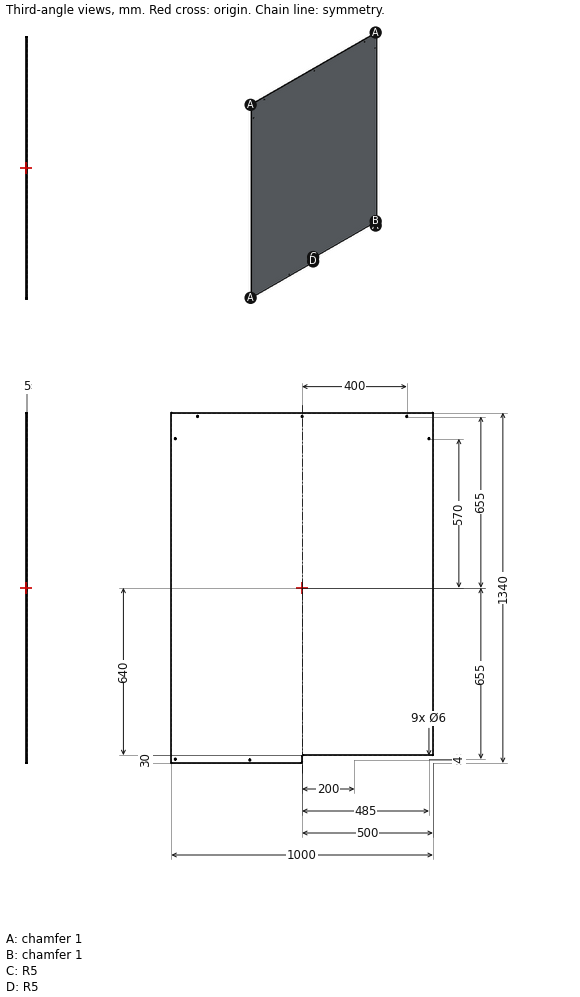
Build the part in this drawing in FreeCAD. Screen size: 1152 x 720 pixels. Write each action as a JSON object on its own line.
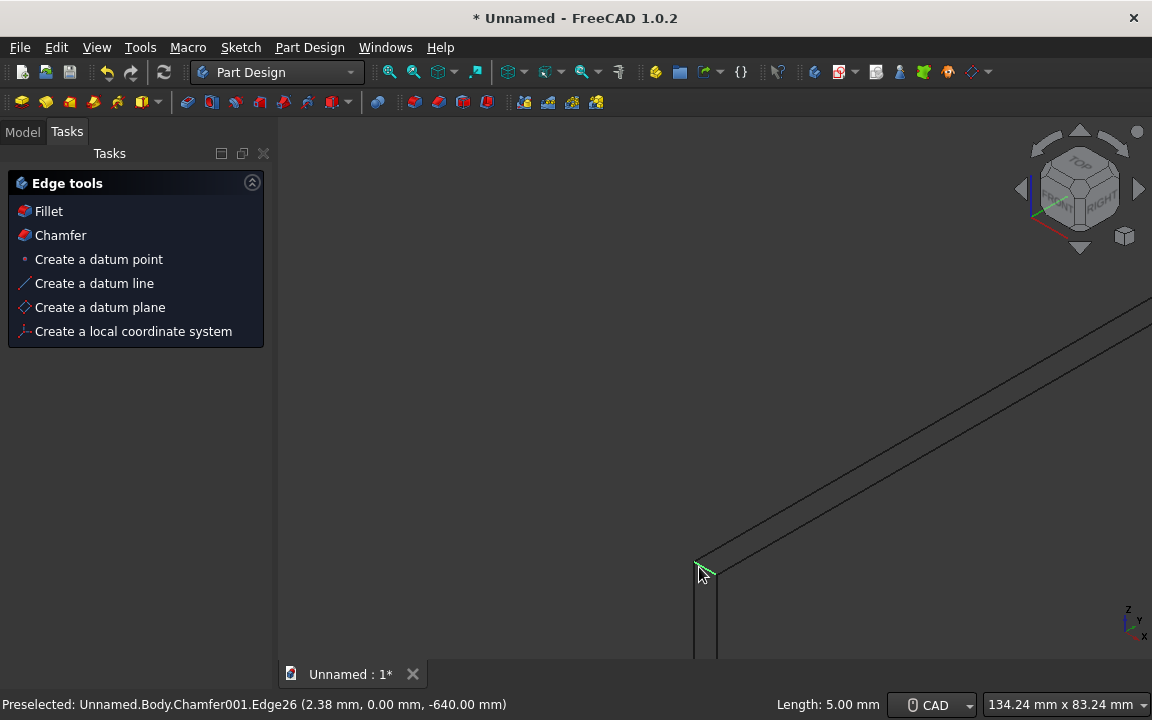
{"action": "key", "text": "v 1"}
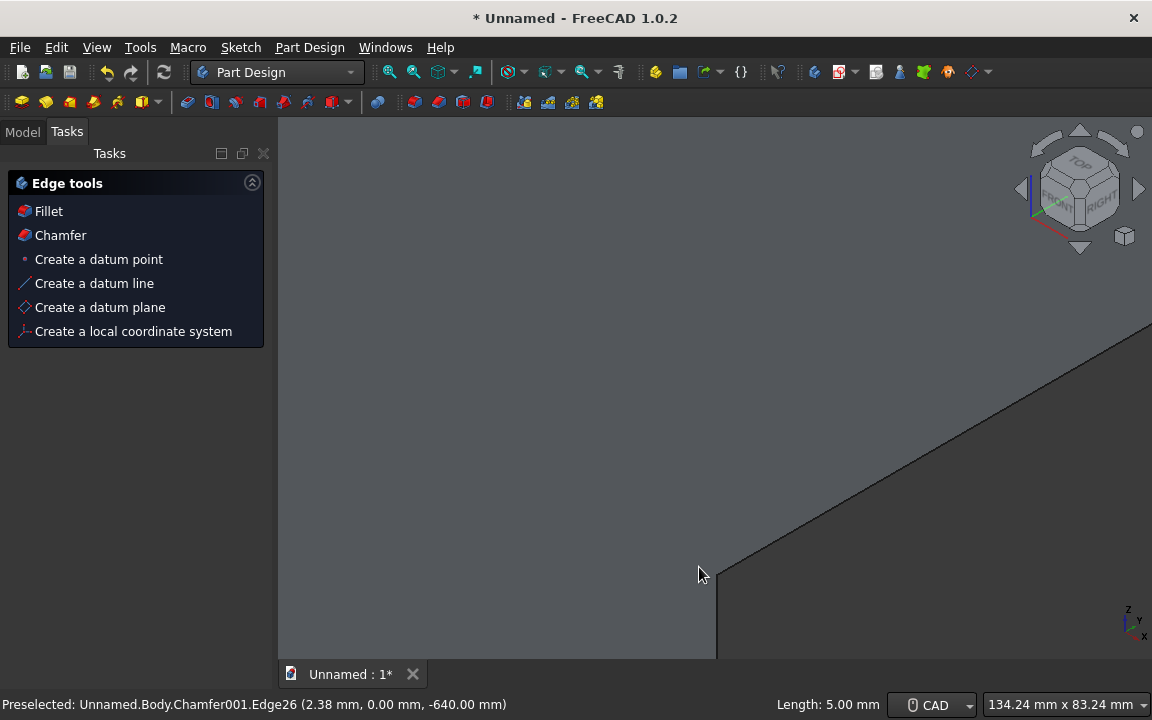
{"action": "left_click", "coordinate": [416, 102]}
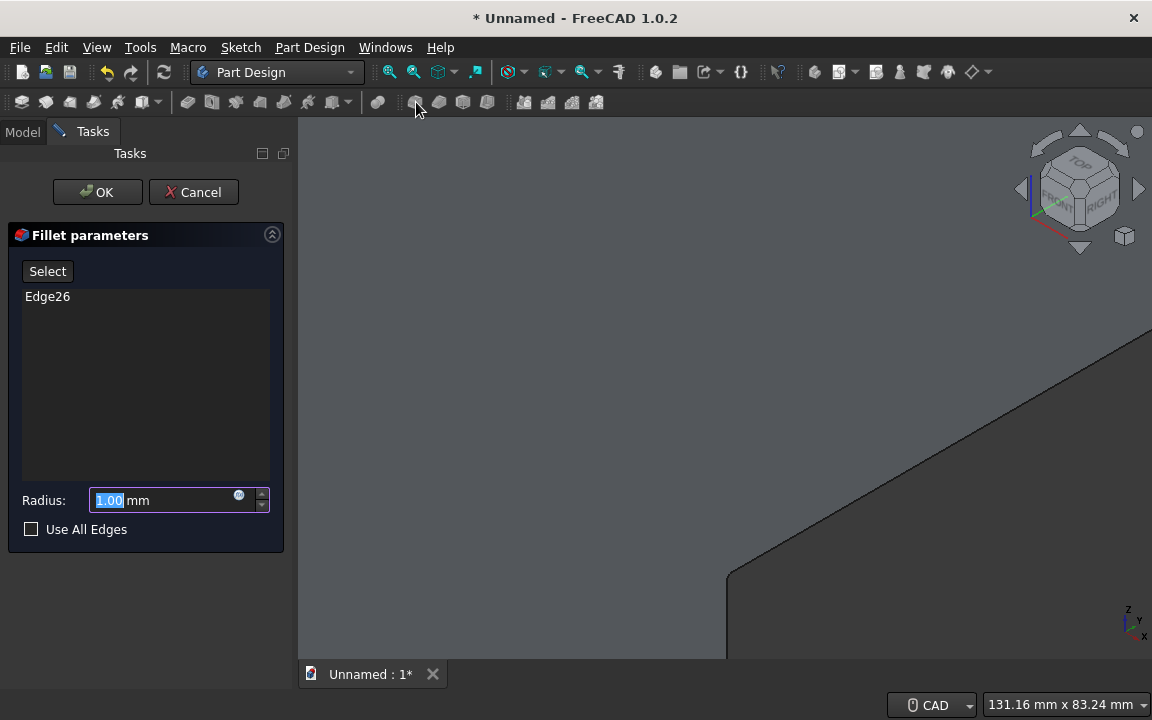
{"action": "type", "text": "5"}
{"action": "key", "text": "Tab"}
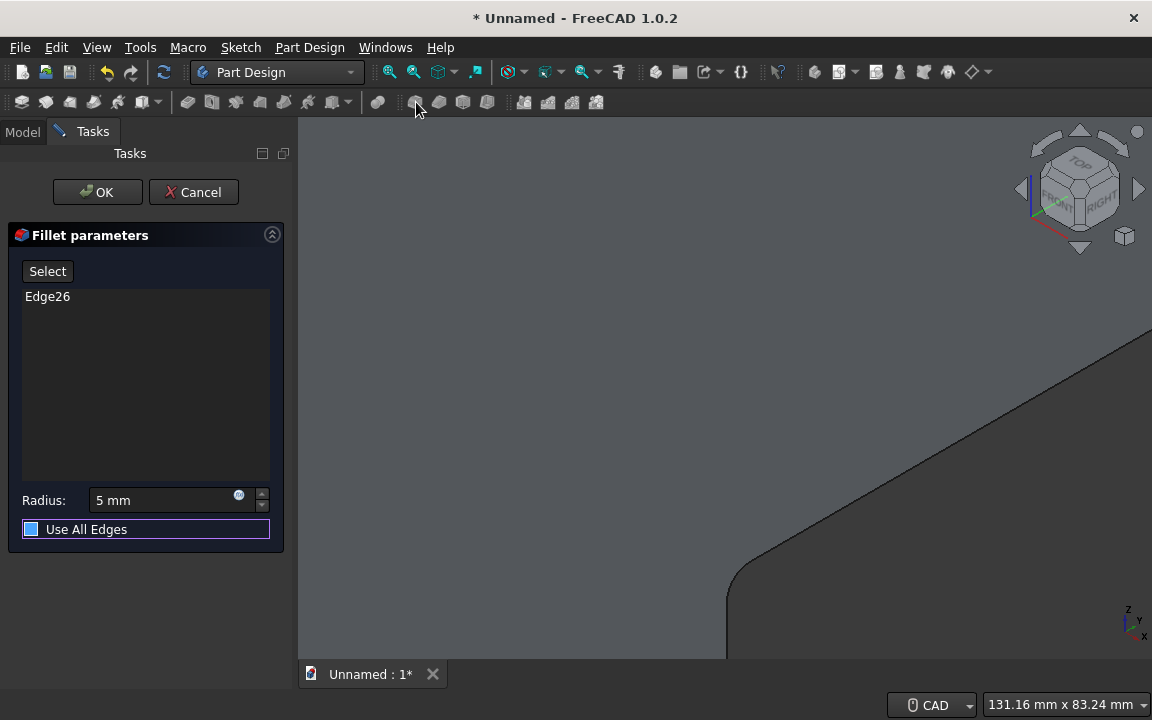
{"action": "left_click", "coordinate": [98, 192]}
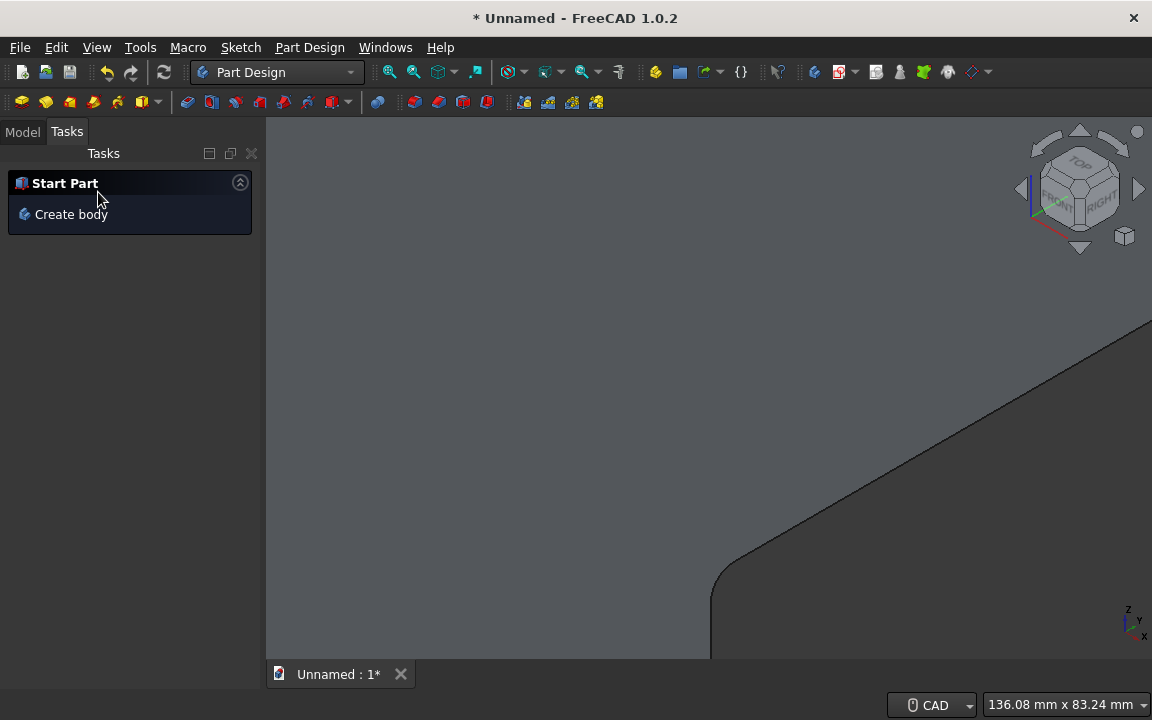
{"action": "left_click", "coordinate": [390, 72]}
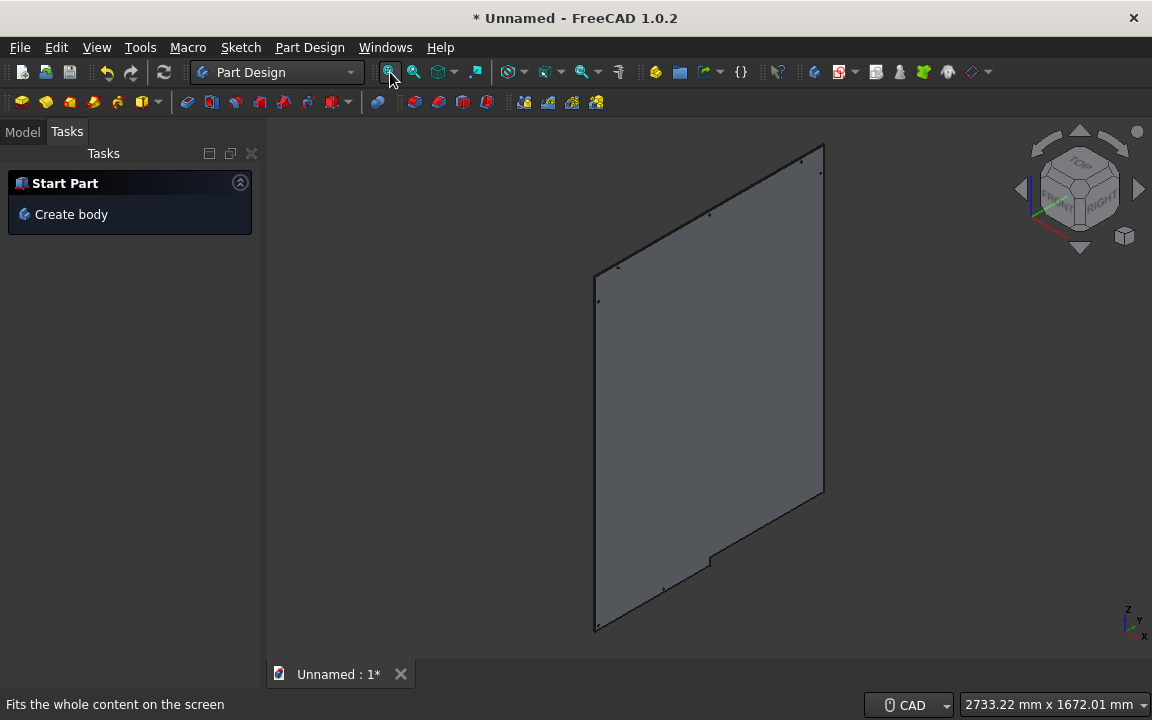
{"action": "scroll", "coordinate": [709, 564], "scroll_direction": "up", "scroll_amount": 15}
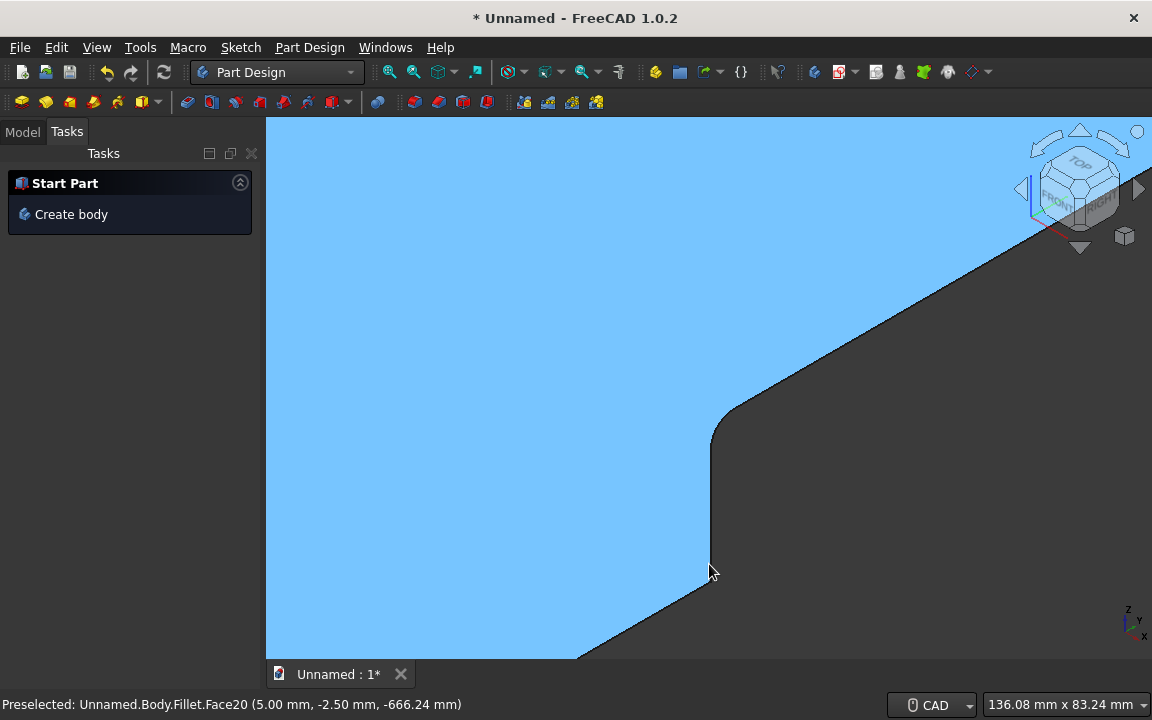
{"action": "left_click", "coordinate": [390, 72]}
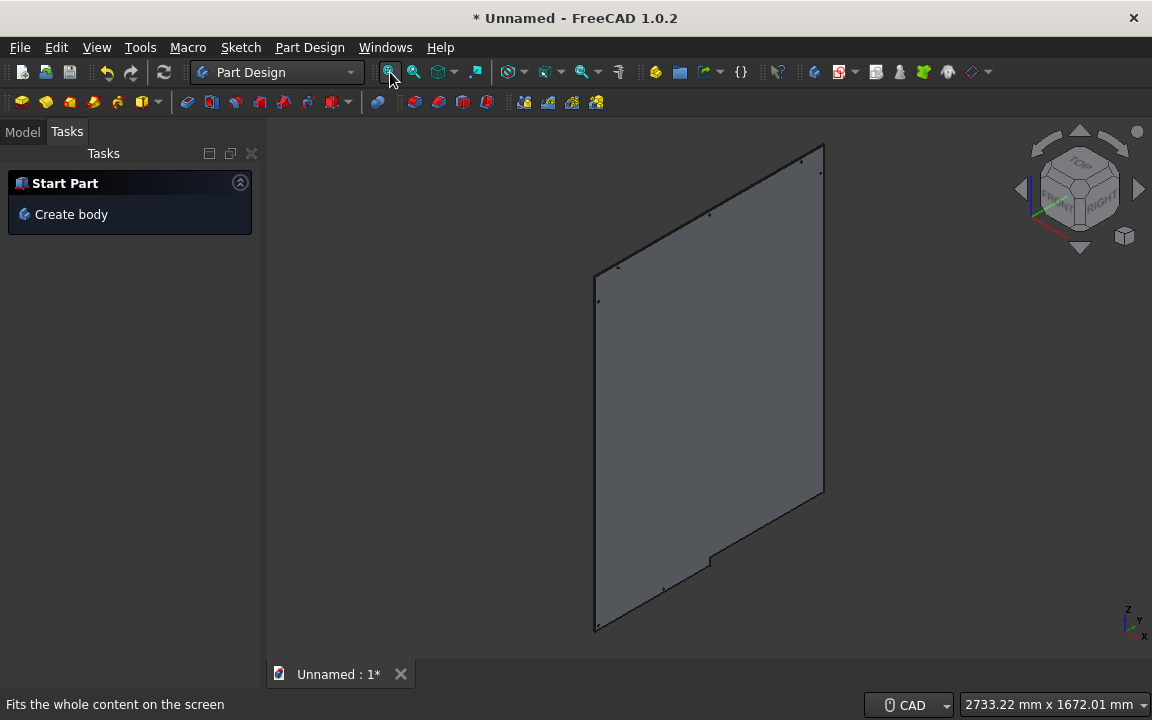
{"action": "key", "text": "2"}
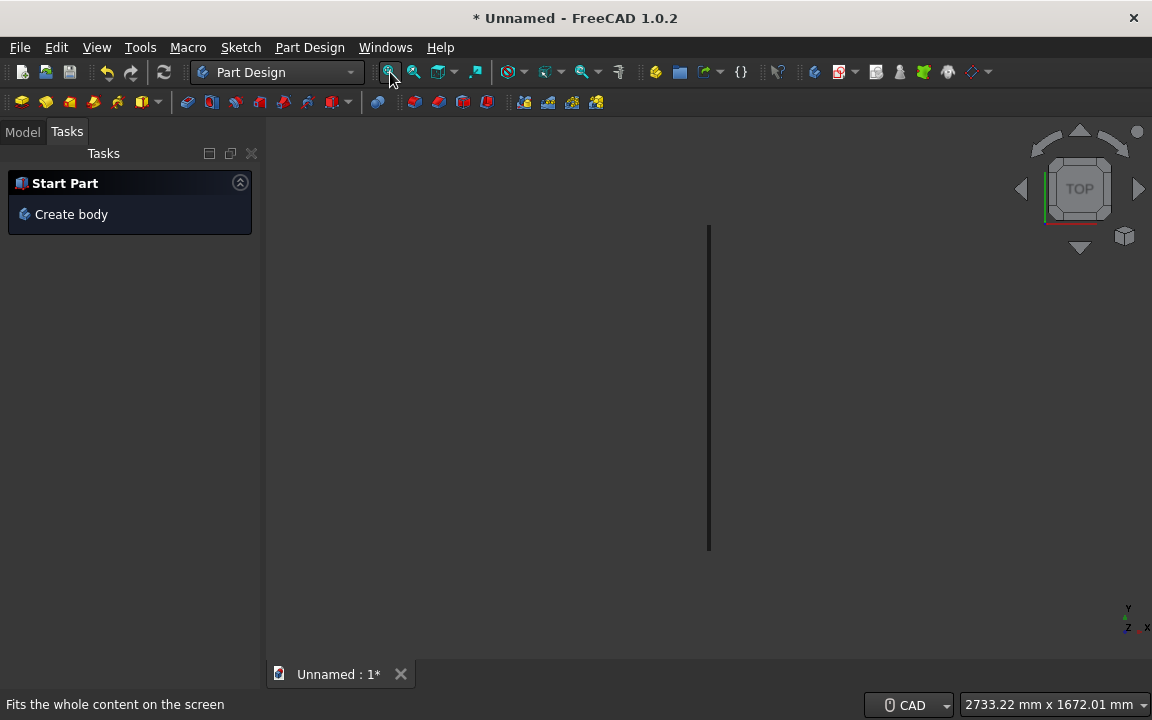
{"action": "scroll", "coordinate": [709, 387], "scroll_direction": "up", "scroll_amount": 15}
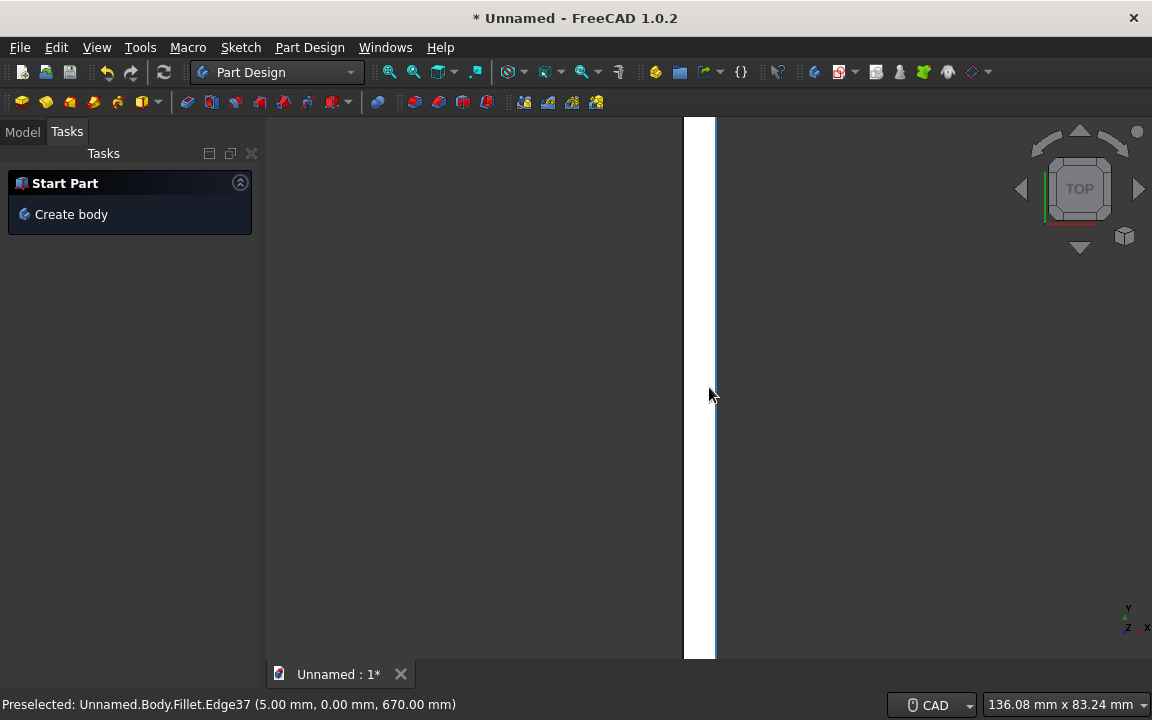
{"action": "left_click", "coordinate": [390, 72]}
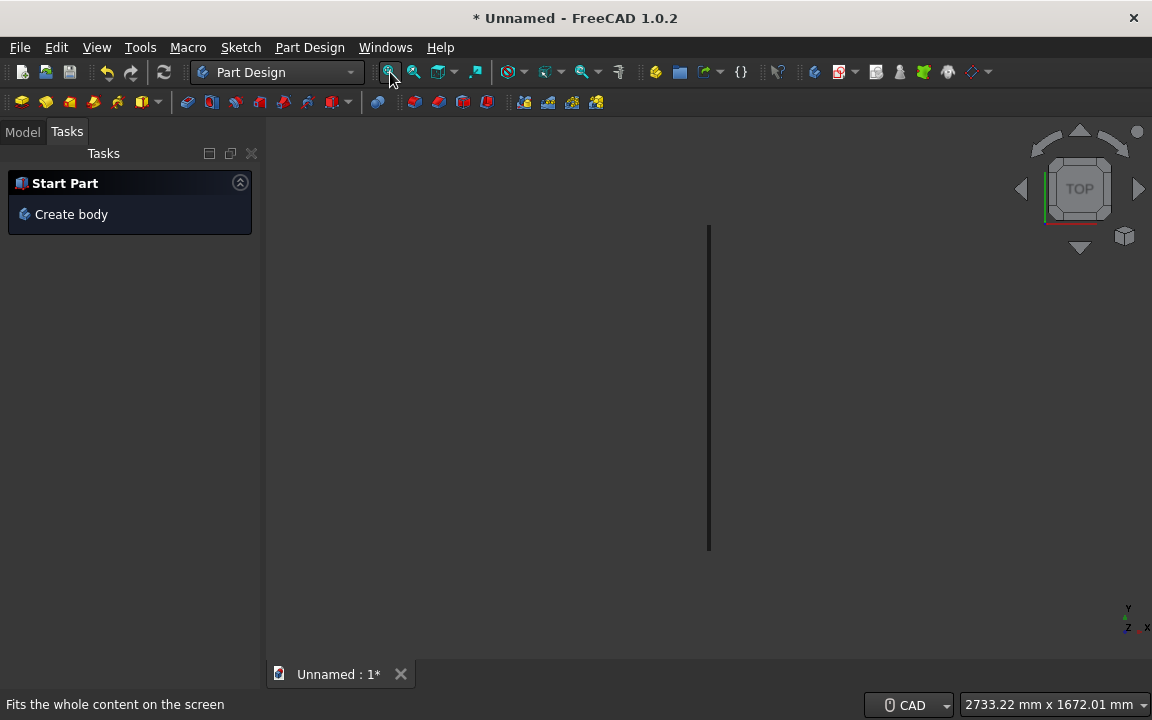
{"action": "key", "text": "0"}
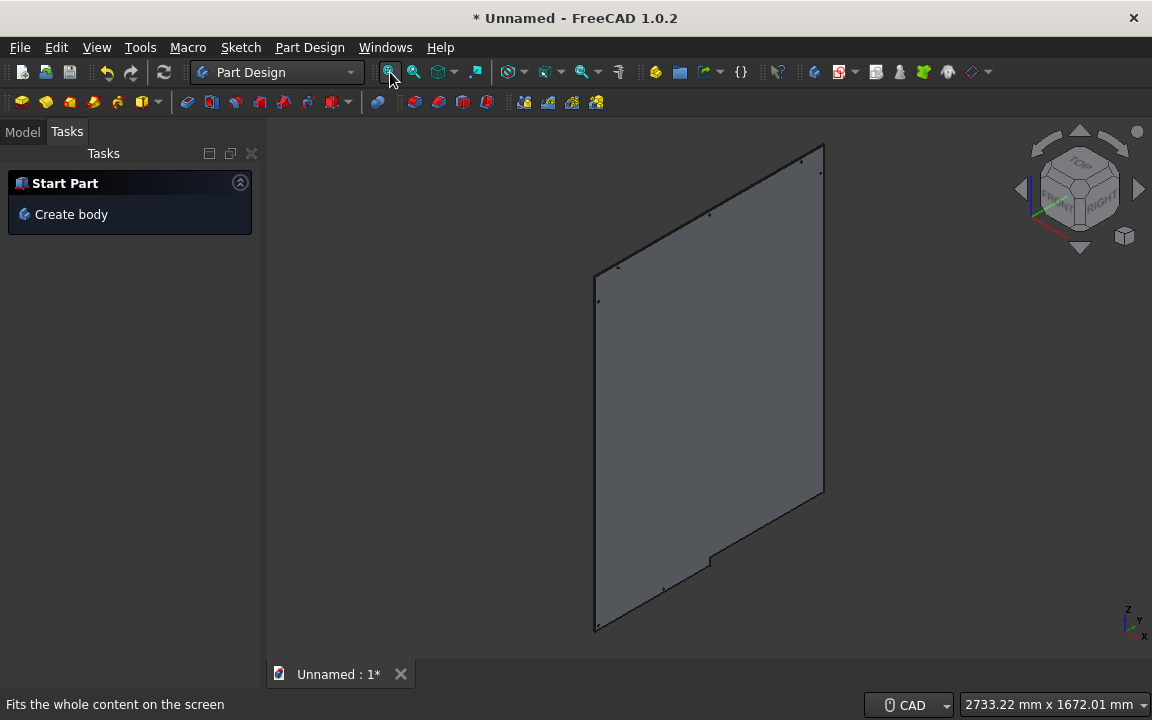
{"action": "scroll", "coordinate": [709, 564], "scroll_direction": "up", "scroll_amount": 15}